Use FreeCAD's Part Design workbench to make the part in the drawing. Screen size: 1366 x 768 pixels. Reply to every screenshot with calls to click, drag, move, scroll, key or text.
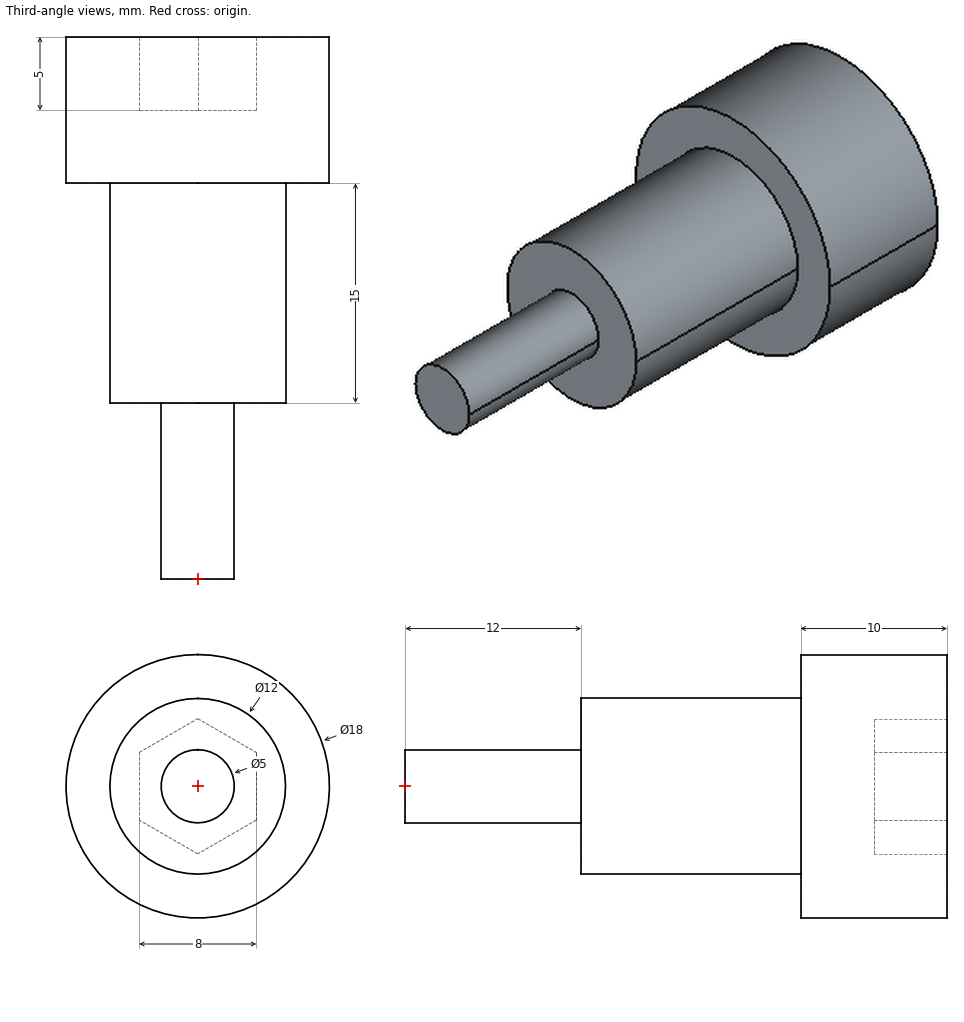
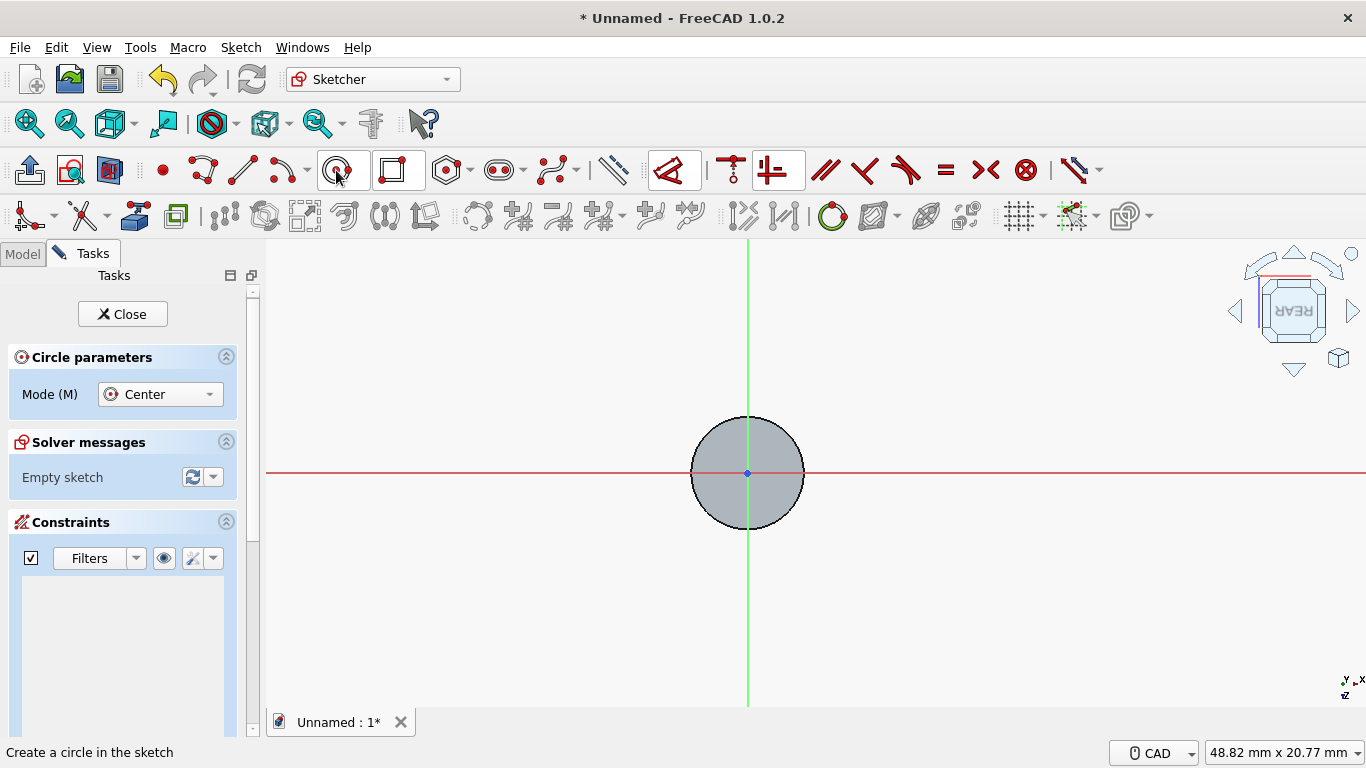
click(748, 473)
move(843, 378)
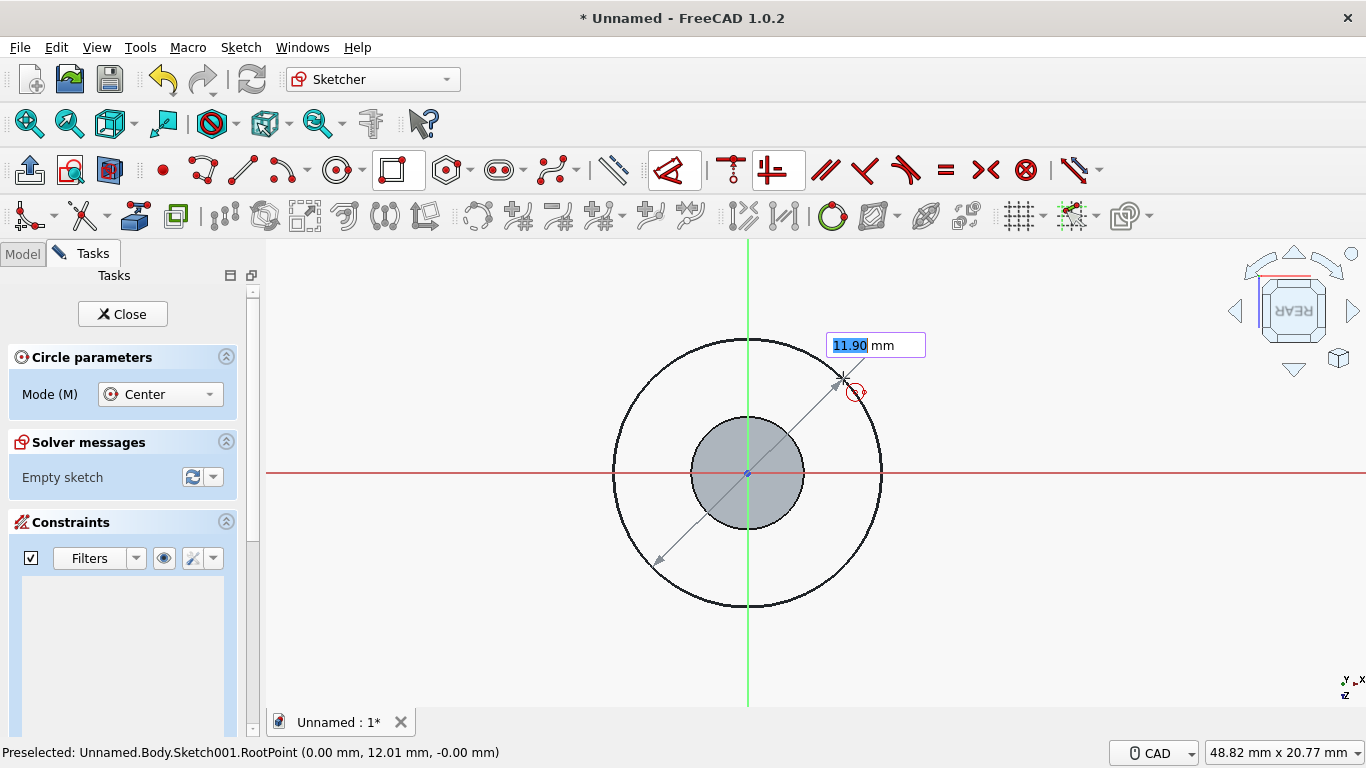
text(12)
key(Return)
key(Escape)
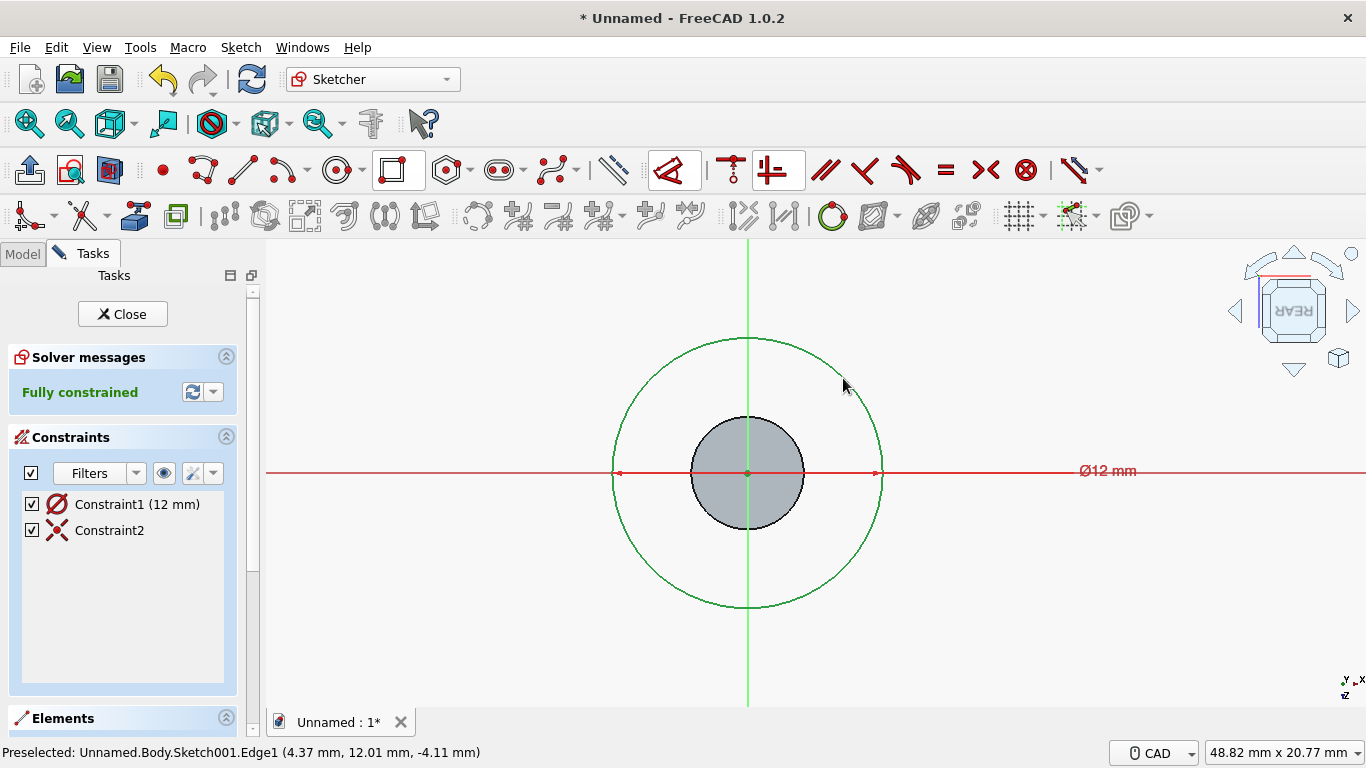
click(123, 314)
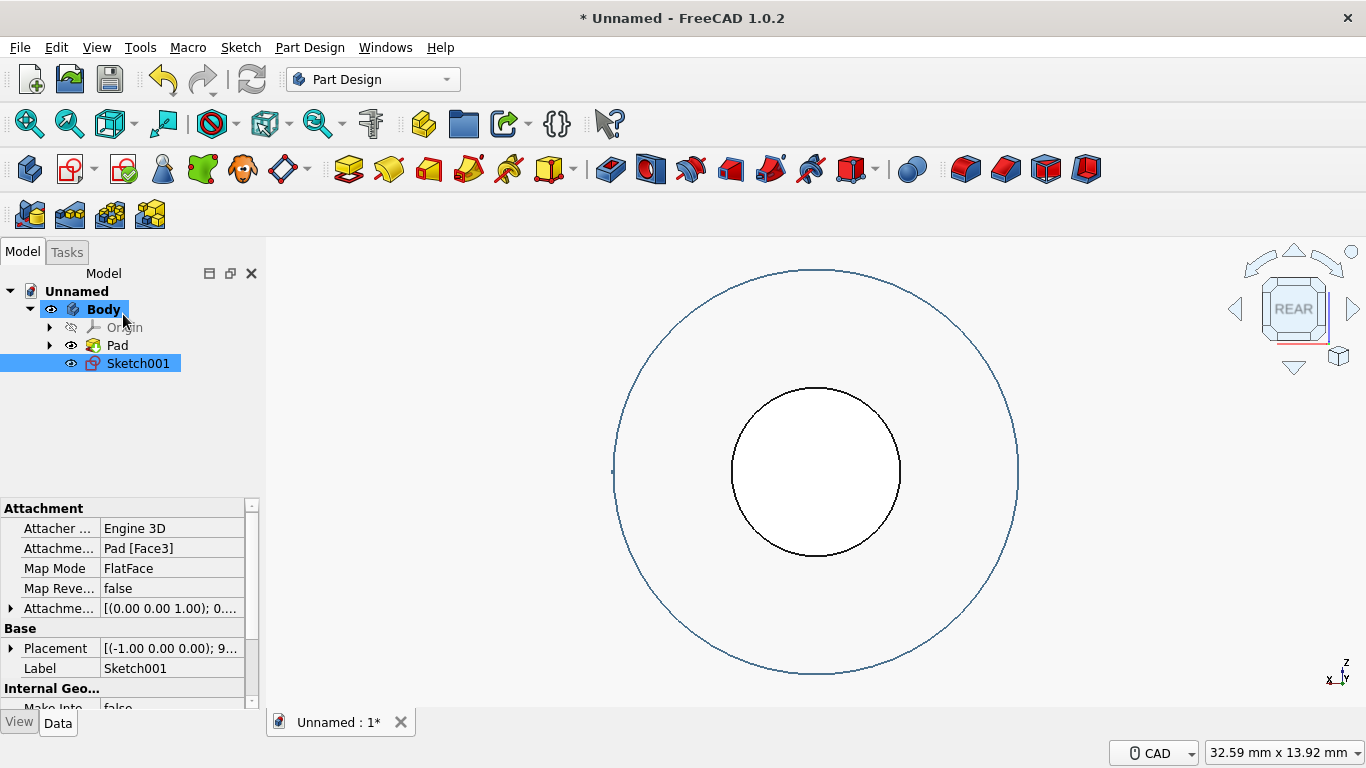
click(350, 170)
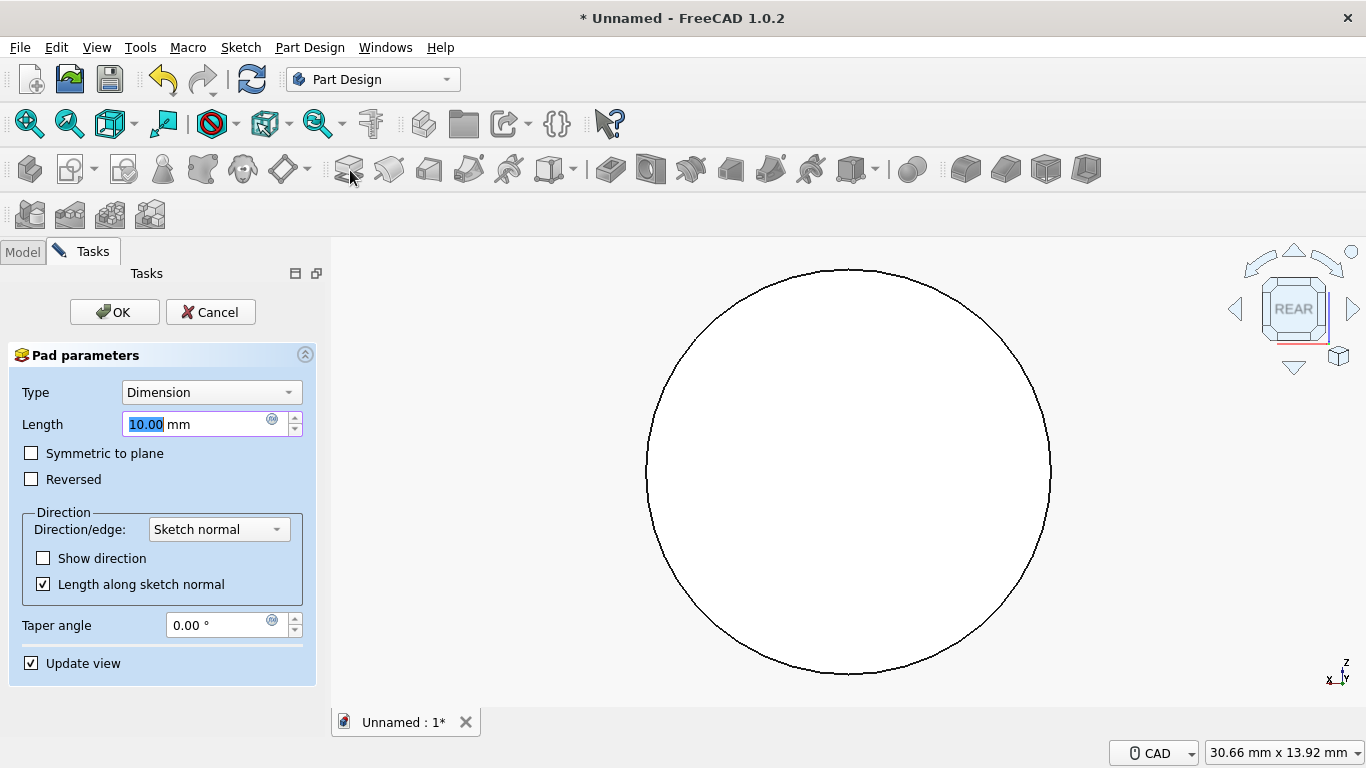
text(15)
key(Tab)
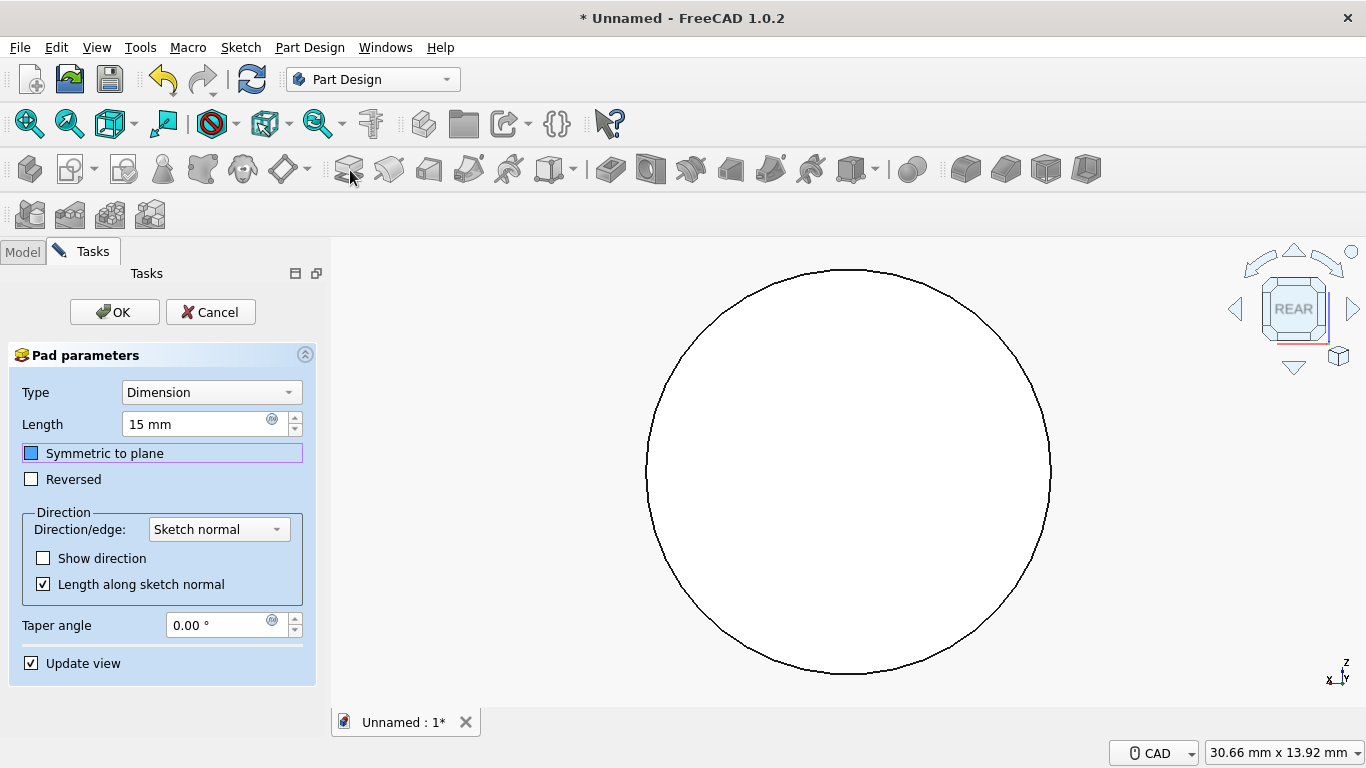
click(115, 312)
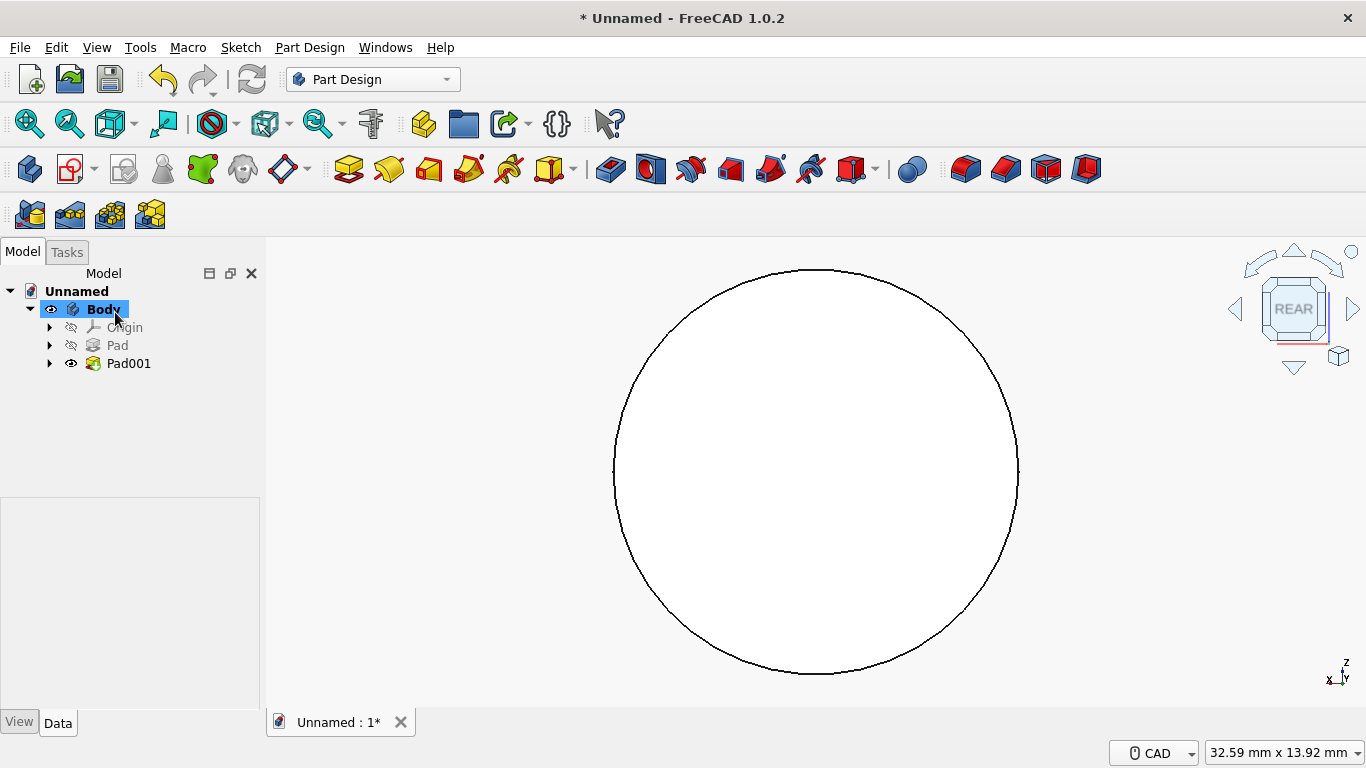
click(816, 471)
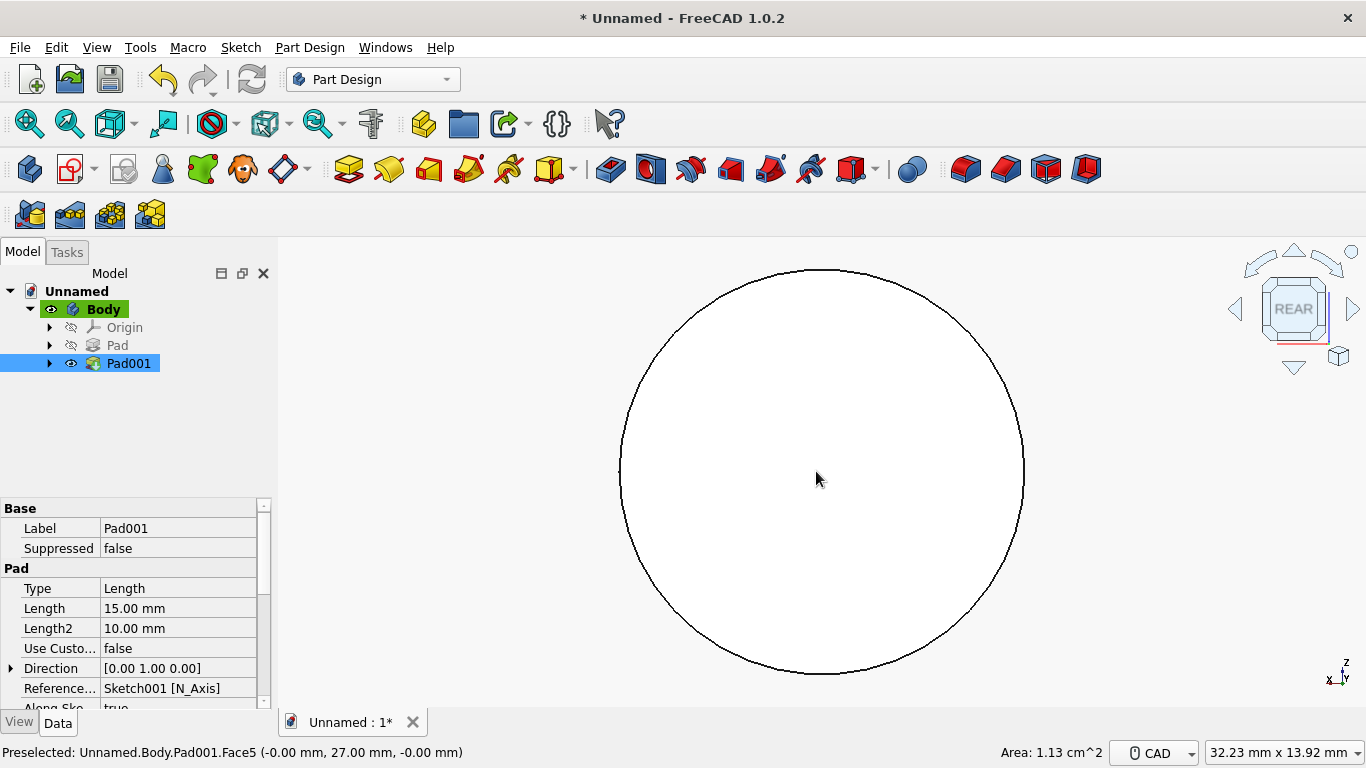
click(70, 170)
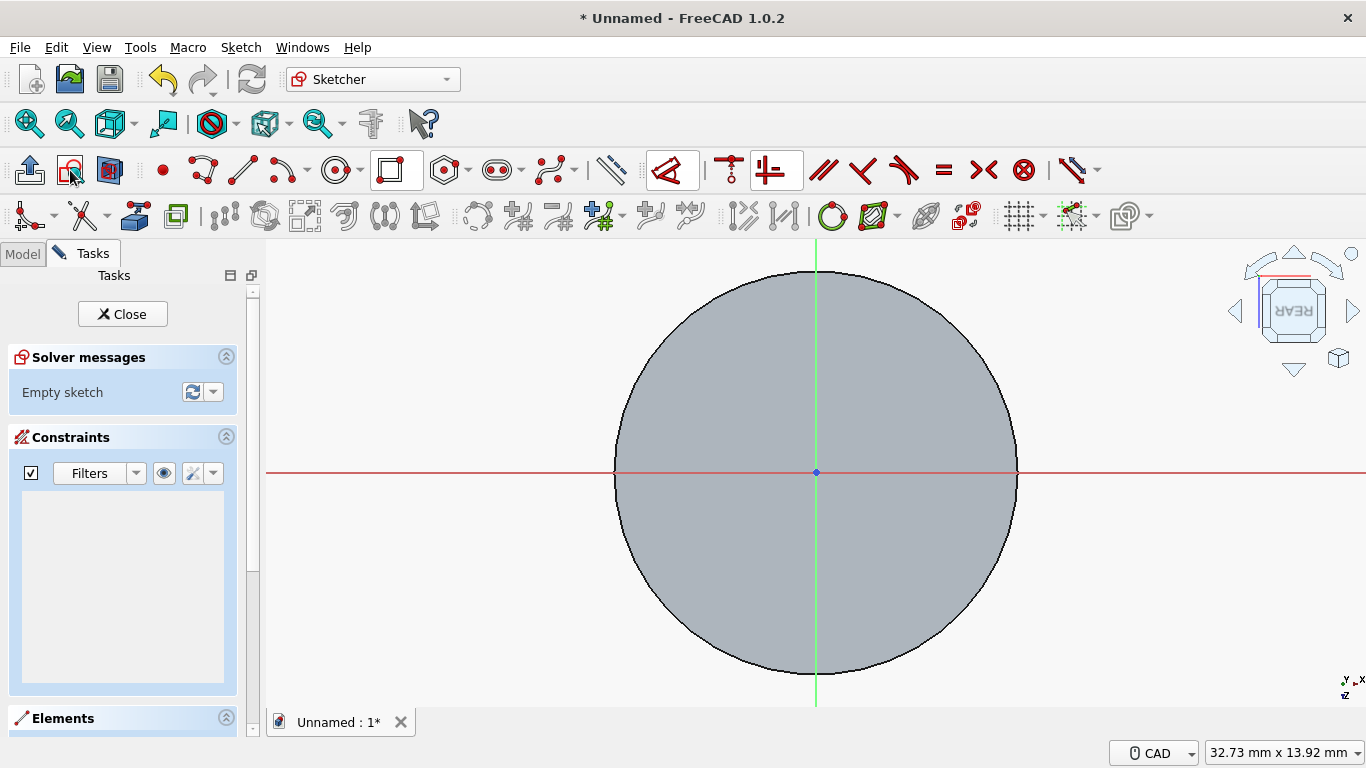
scroll(692, 473, down, 4)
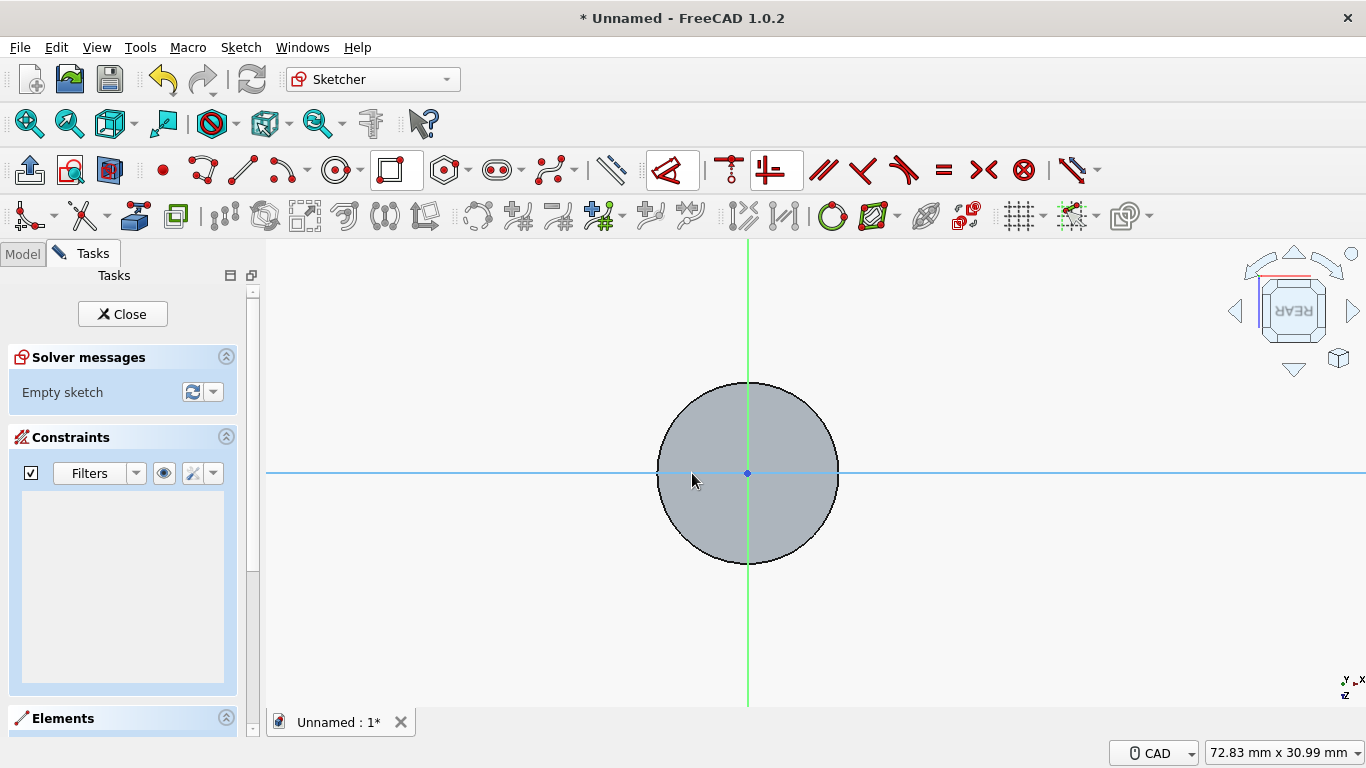
click(336, 170)